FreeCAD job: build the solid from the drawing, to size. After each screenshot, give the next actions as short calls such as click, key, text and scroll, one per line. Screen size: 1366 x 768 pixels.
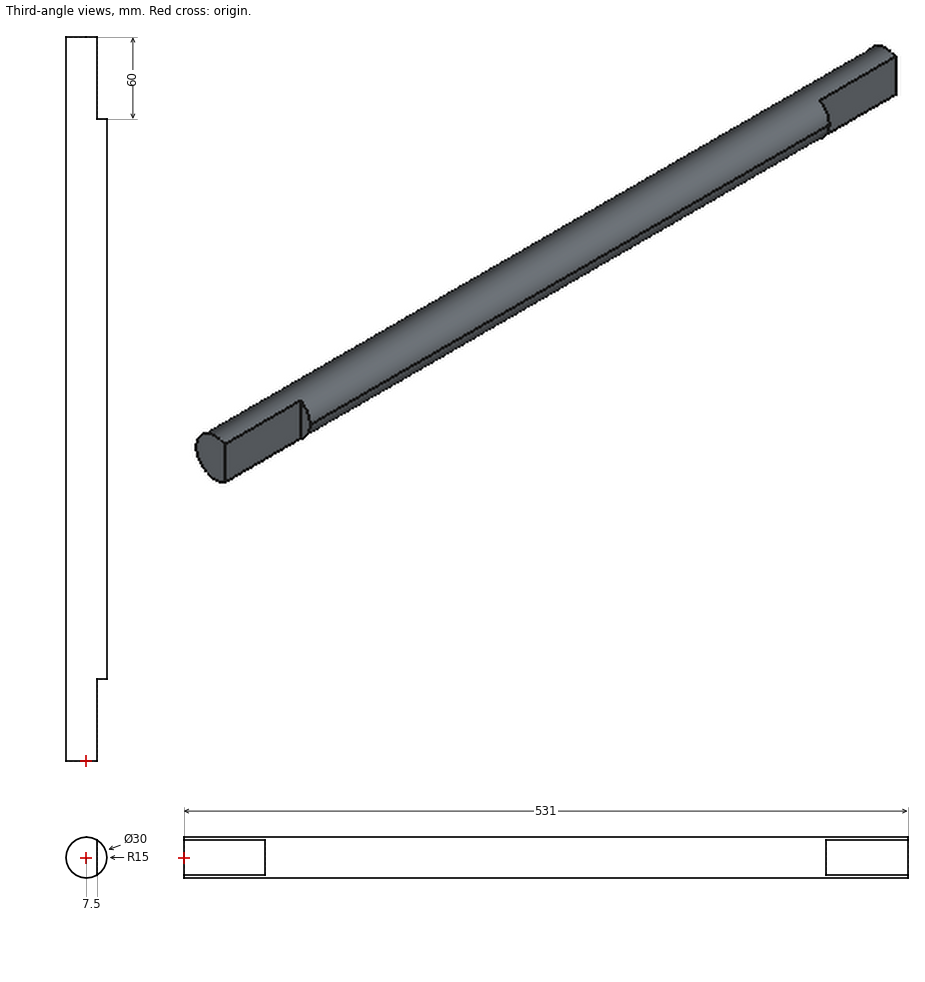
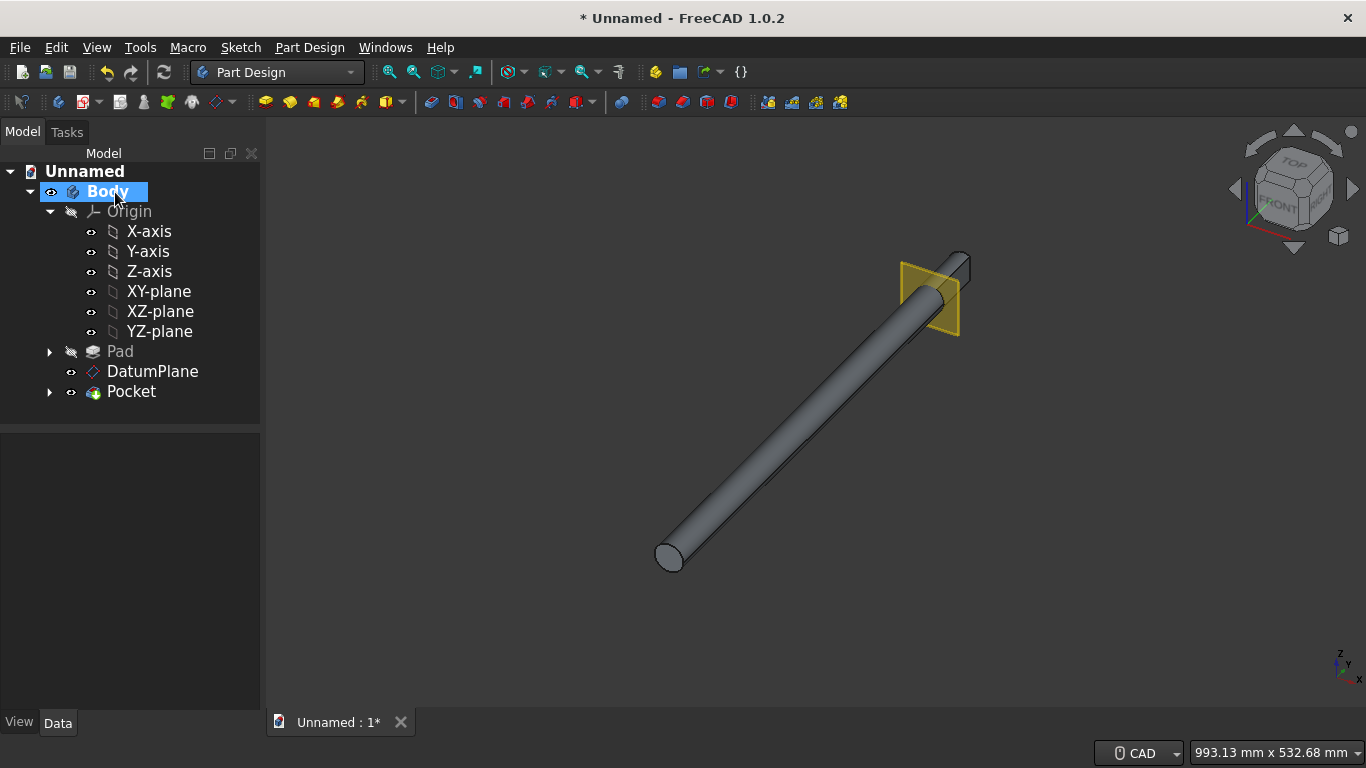
click(116, 372)
key(space)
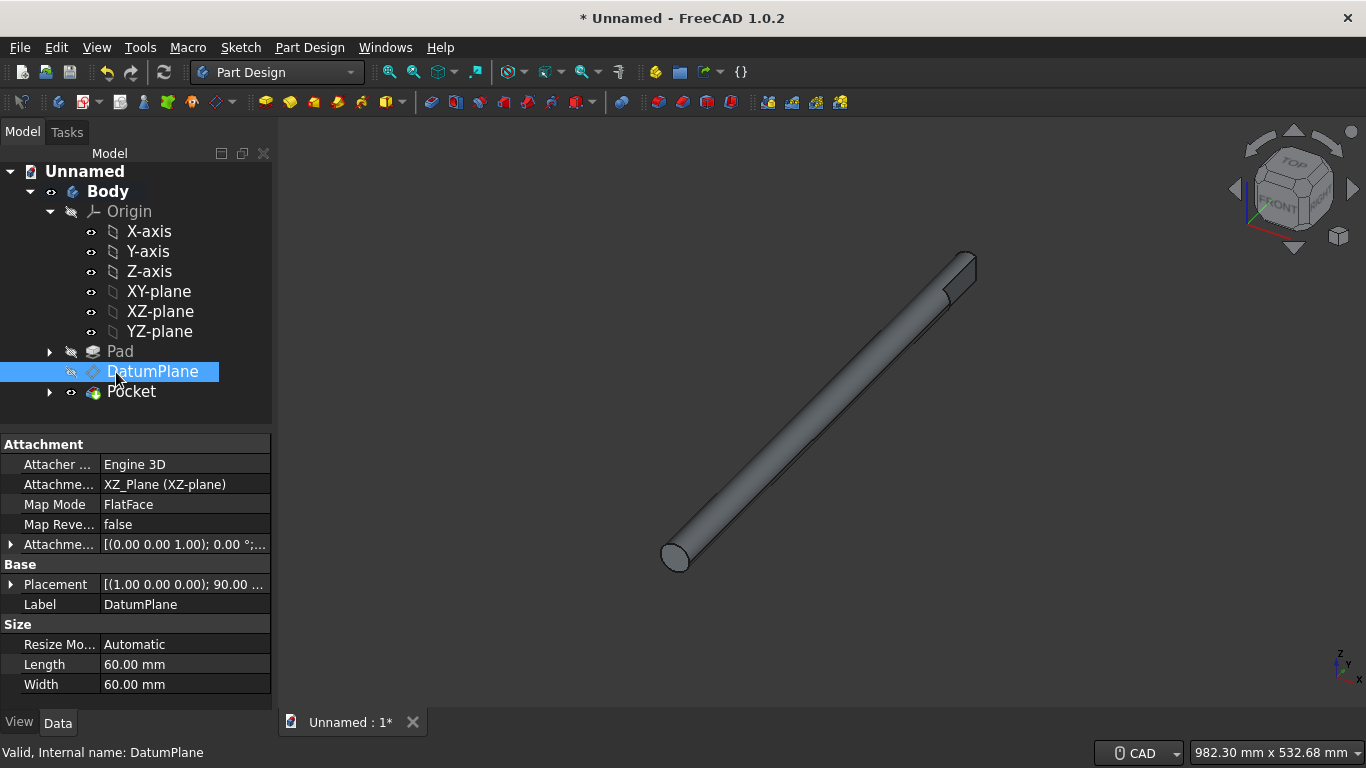
click(136, 312)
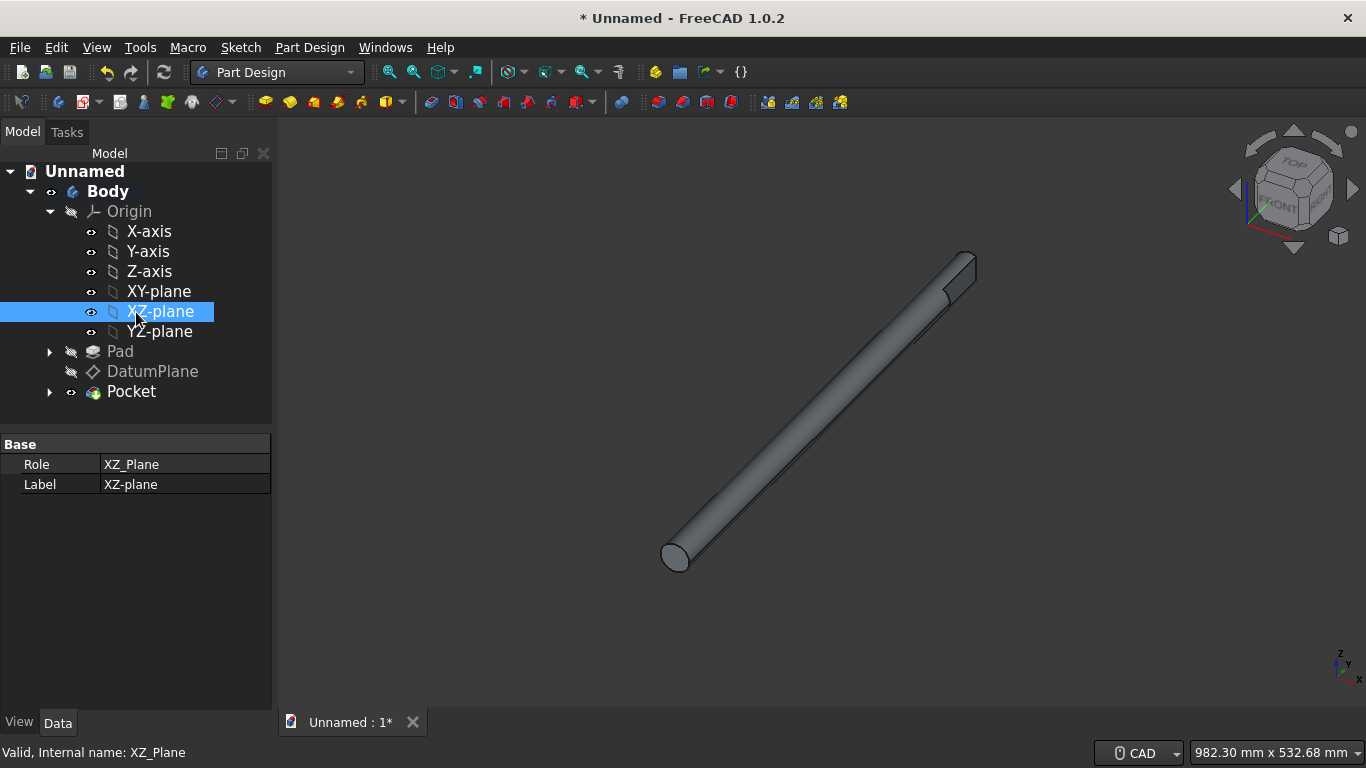
click(216, 102)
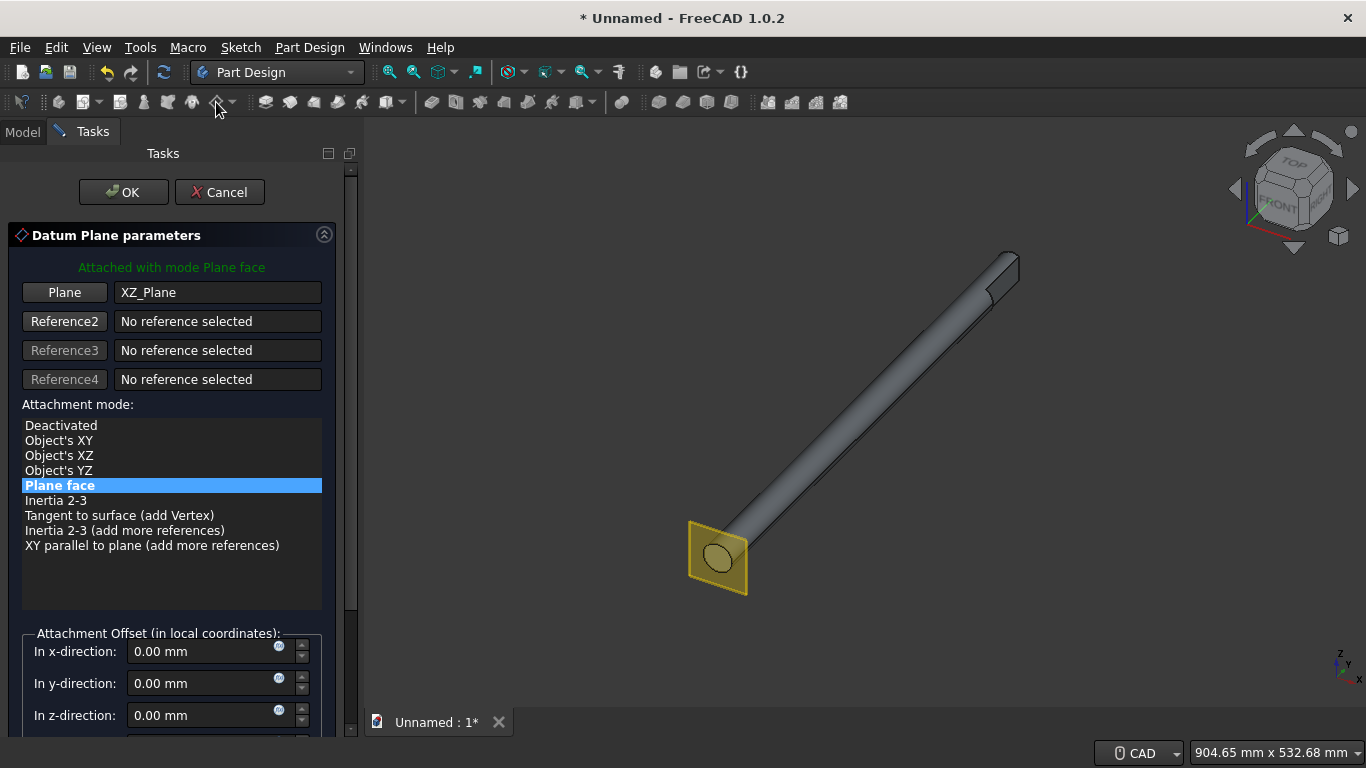
triple_click(210, 715)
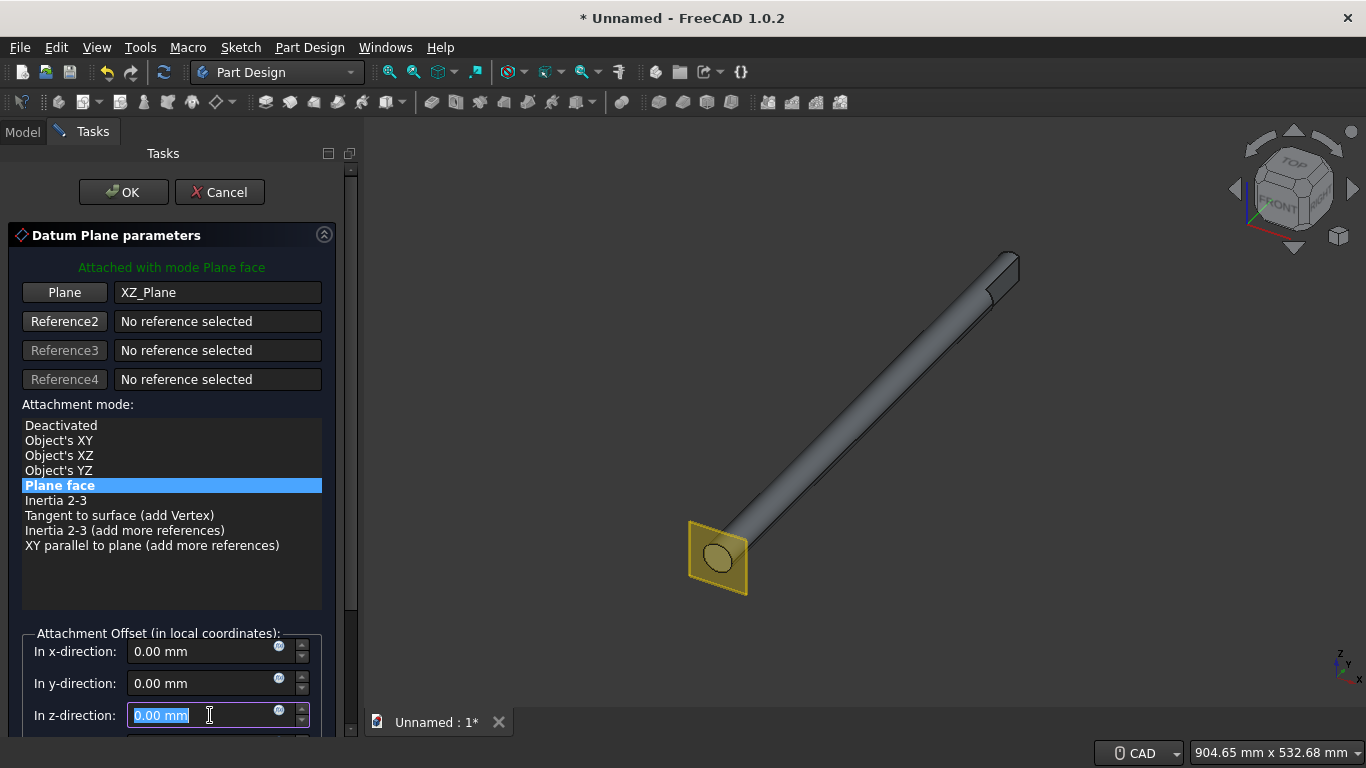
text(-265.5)
key(Tab)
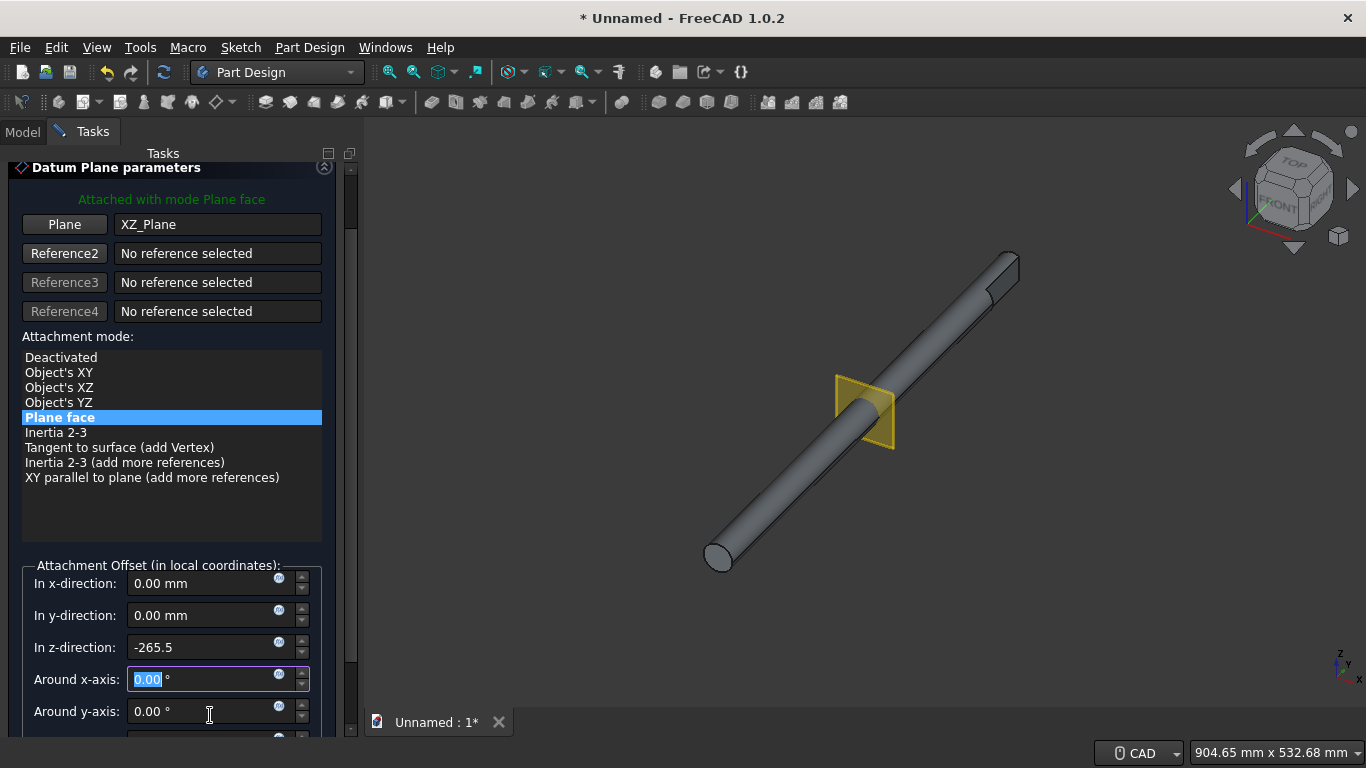
scroll(351, 450, up, 2)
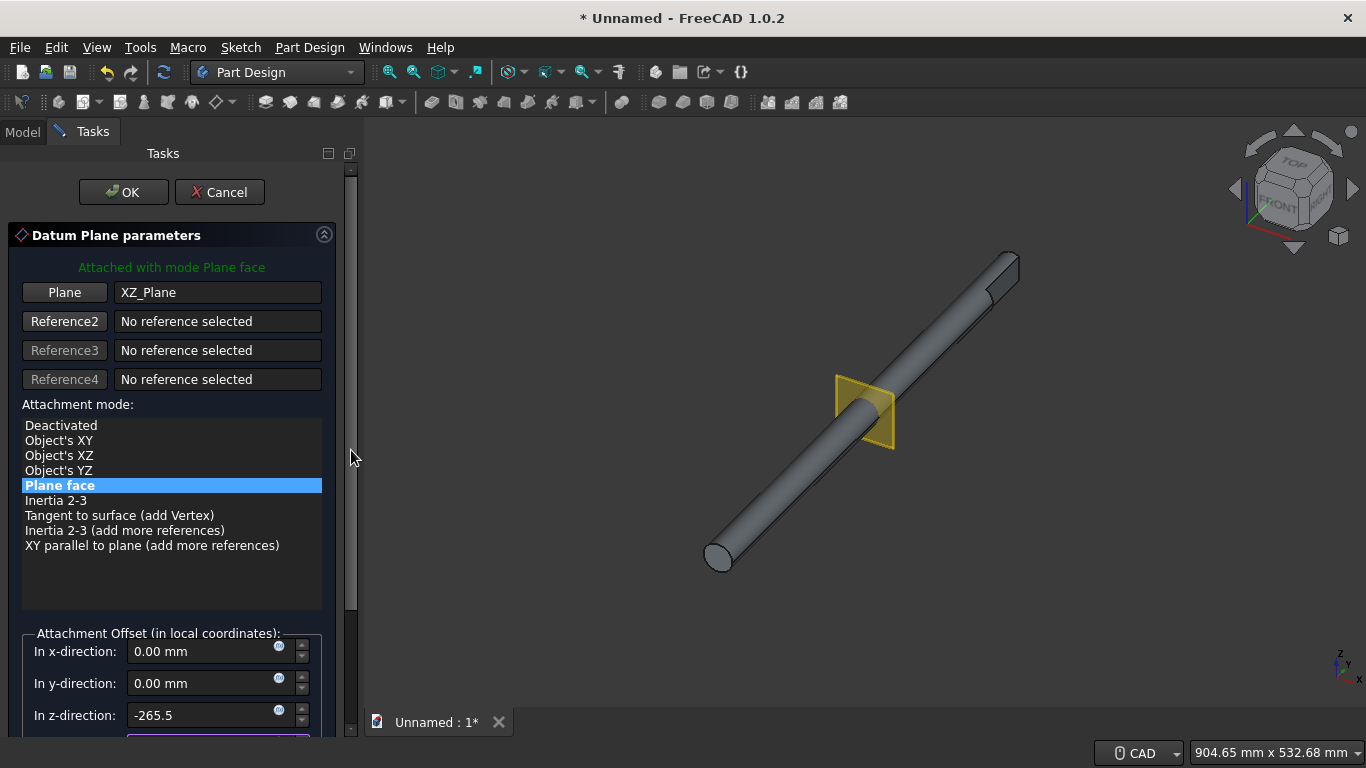
click(124, 192)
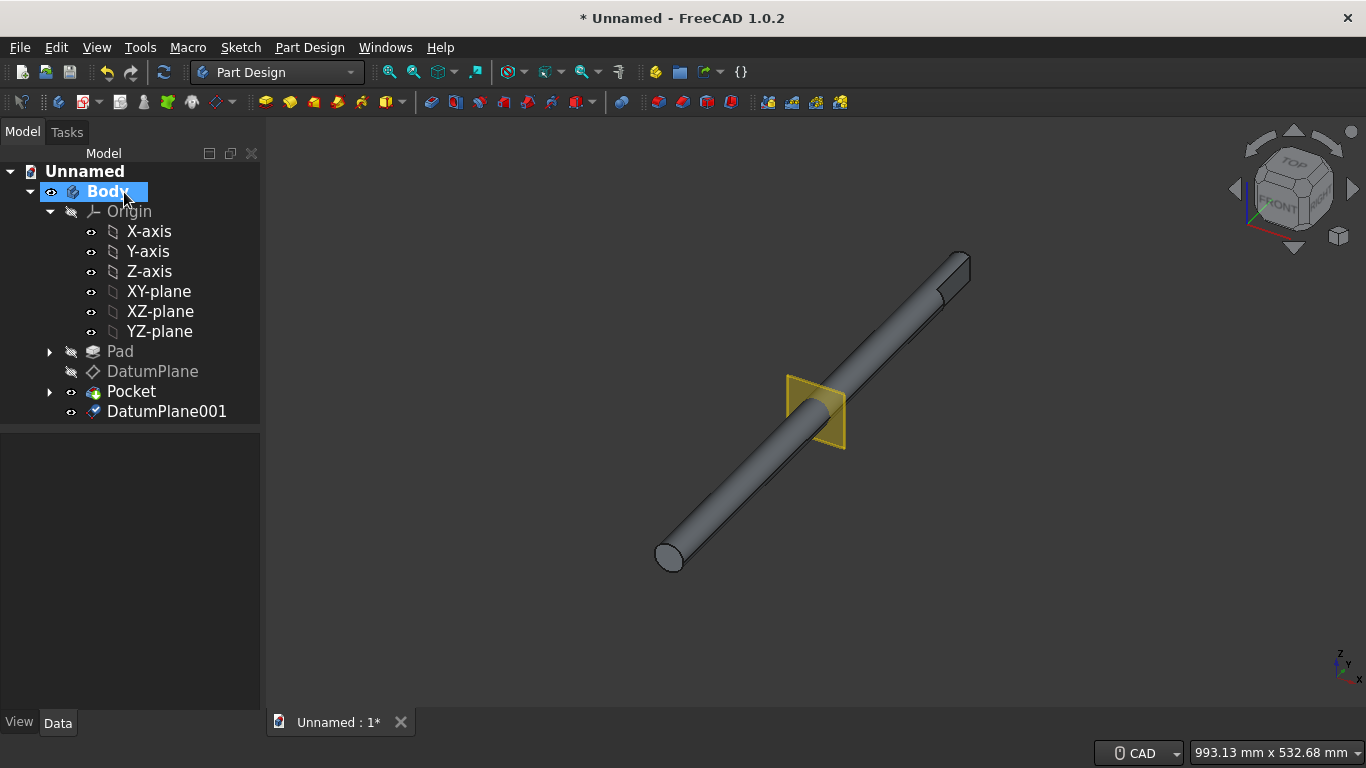
click(116, 392)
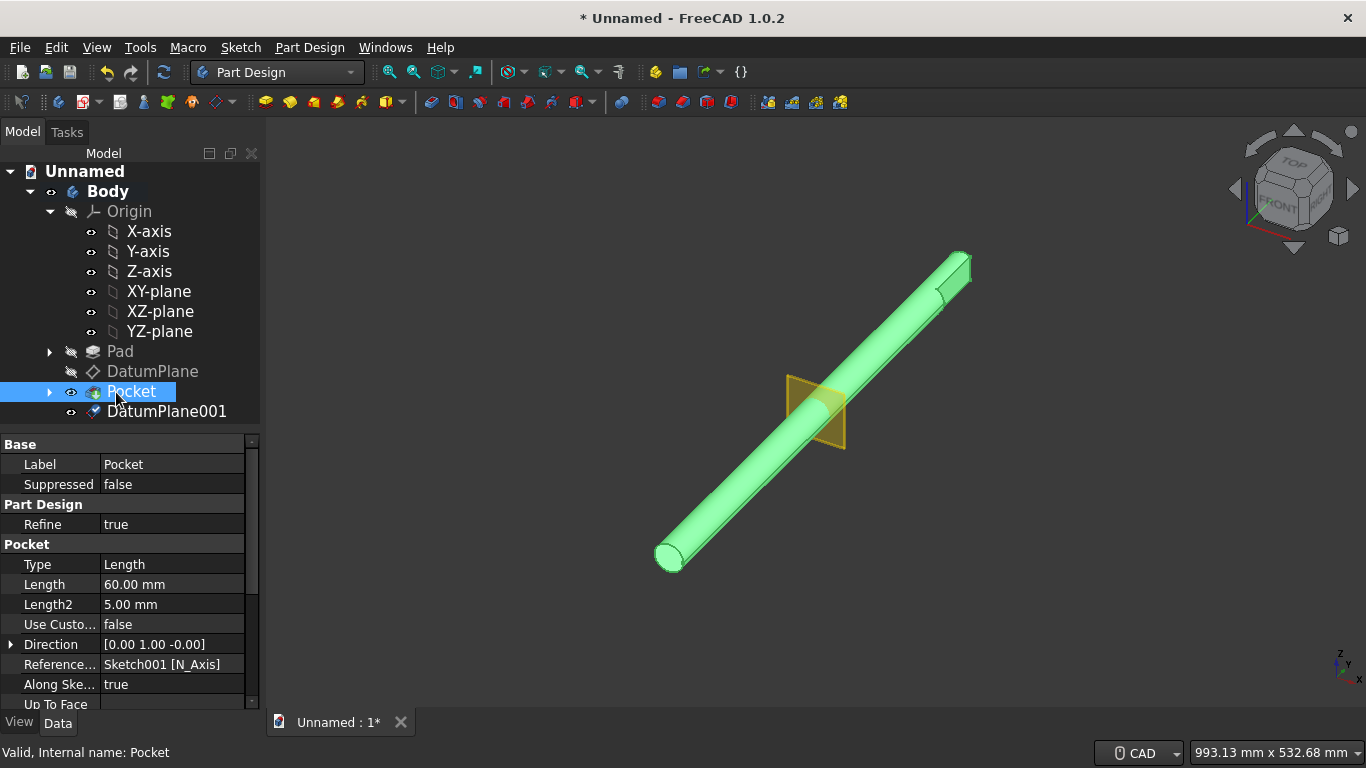
click(768, 102)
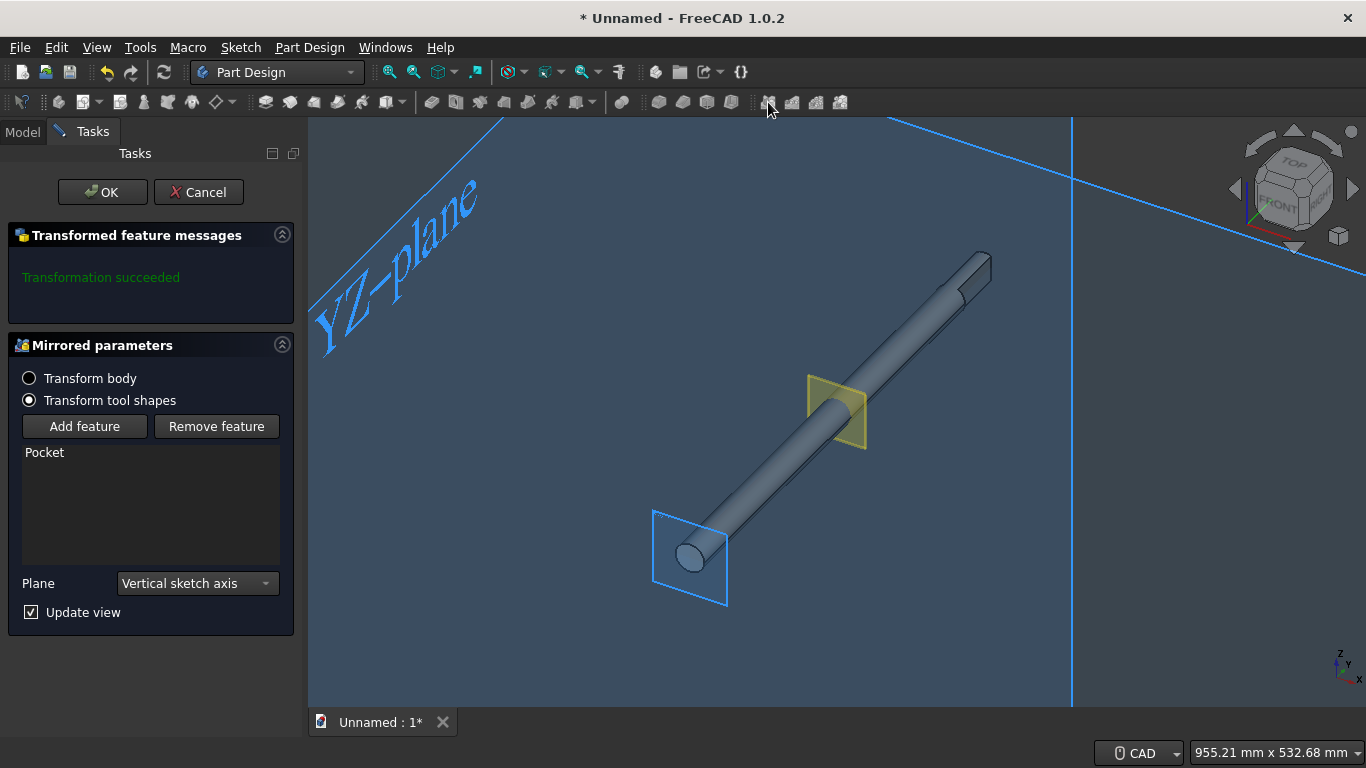
click(198, 584)